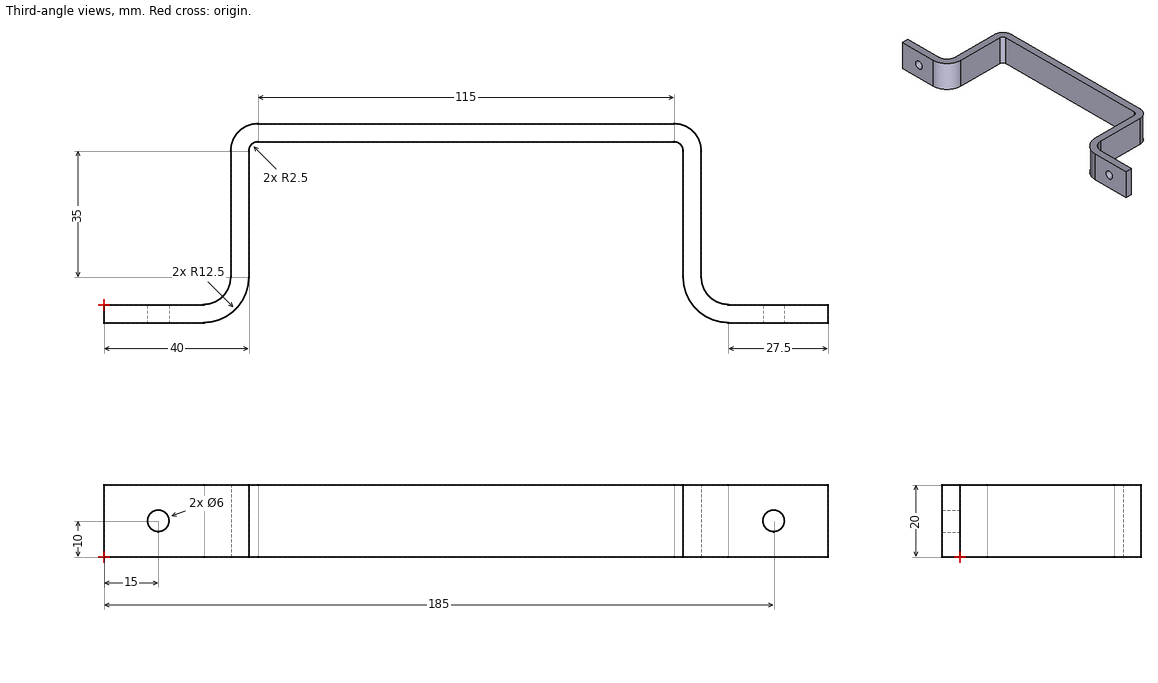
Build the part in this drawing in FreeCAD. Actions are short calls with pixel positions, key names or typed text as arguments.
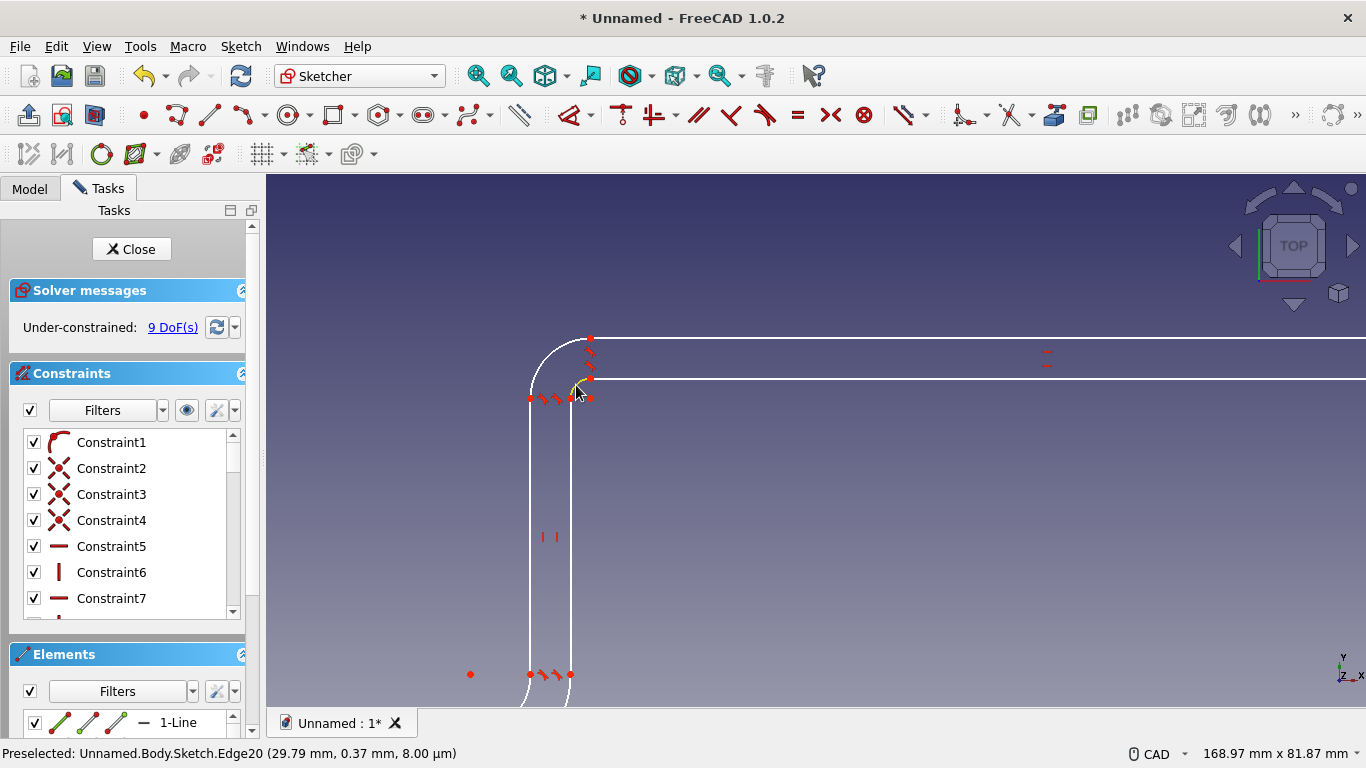
click(576, 384)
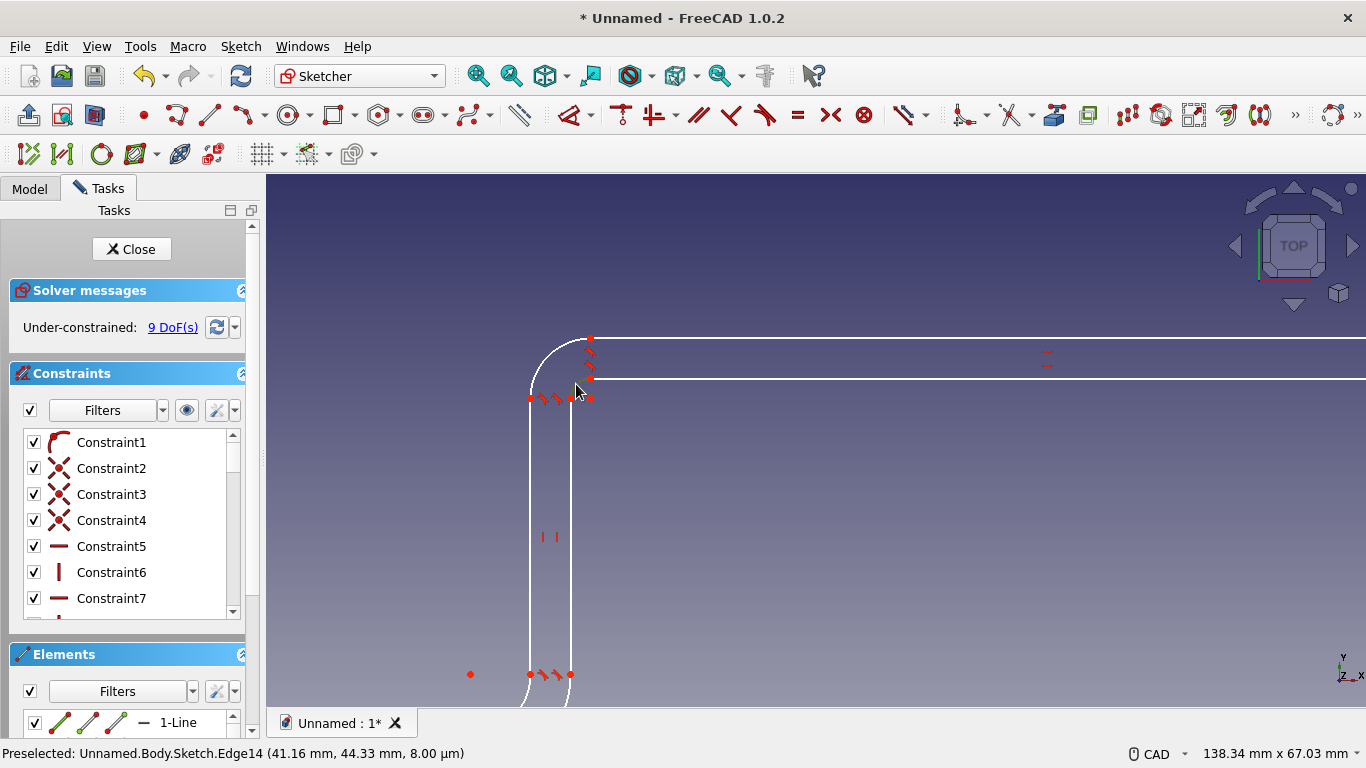
scroll(573, 373, down, 5)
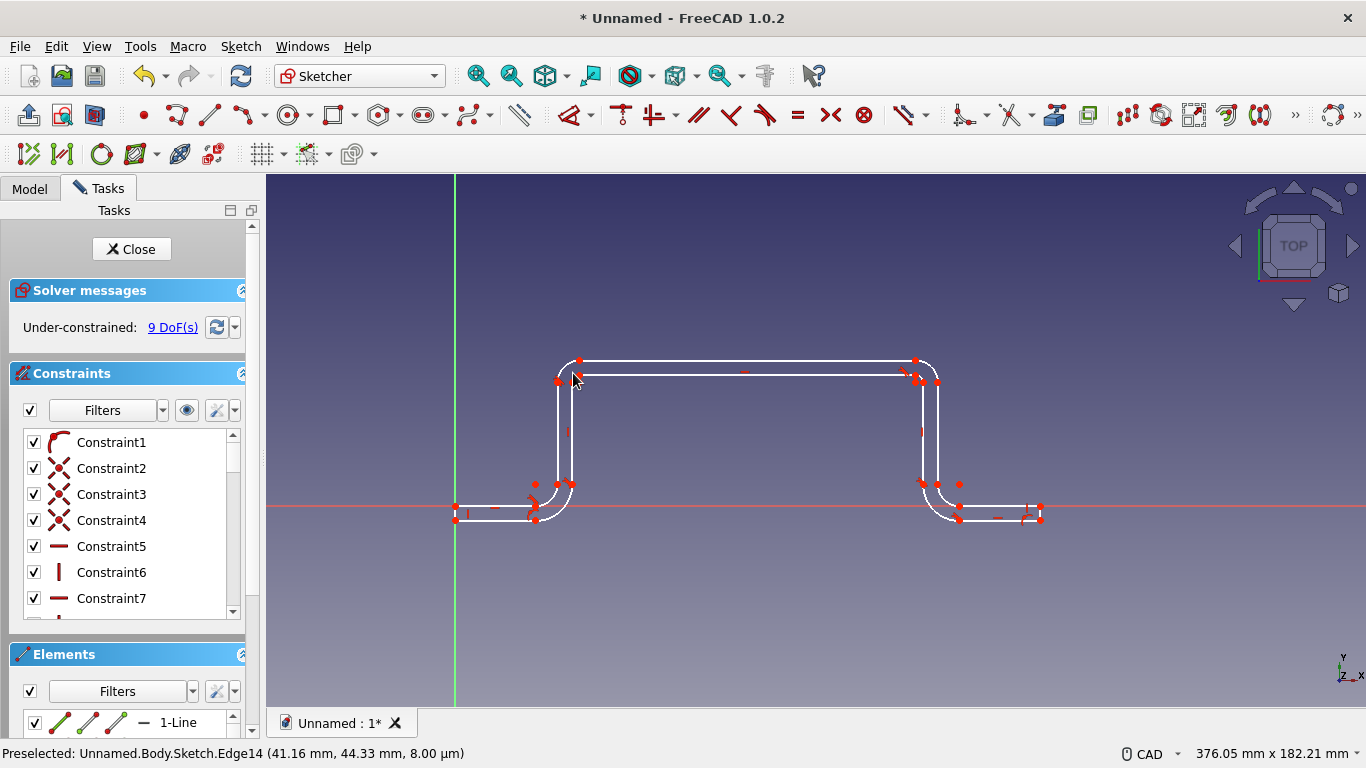
scroll(922, 379, up, 7)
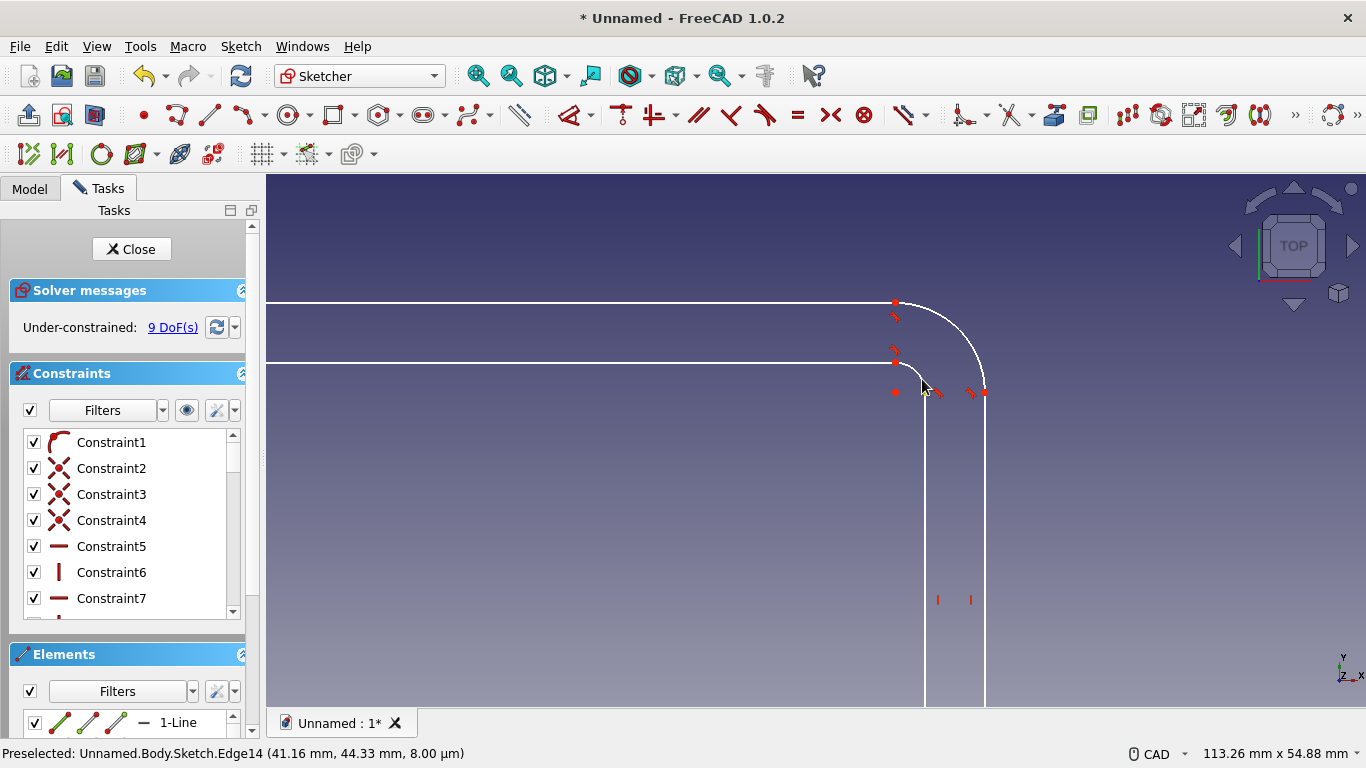
click(922, 379)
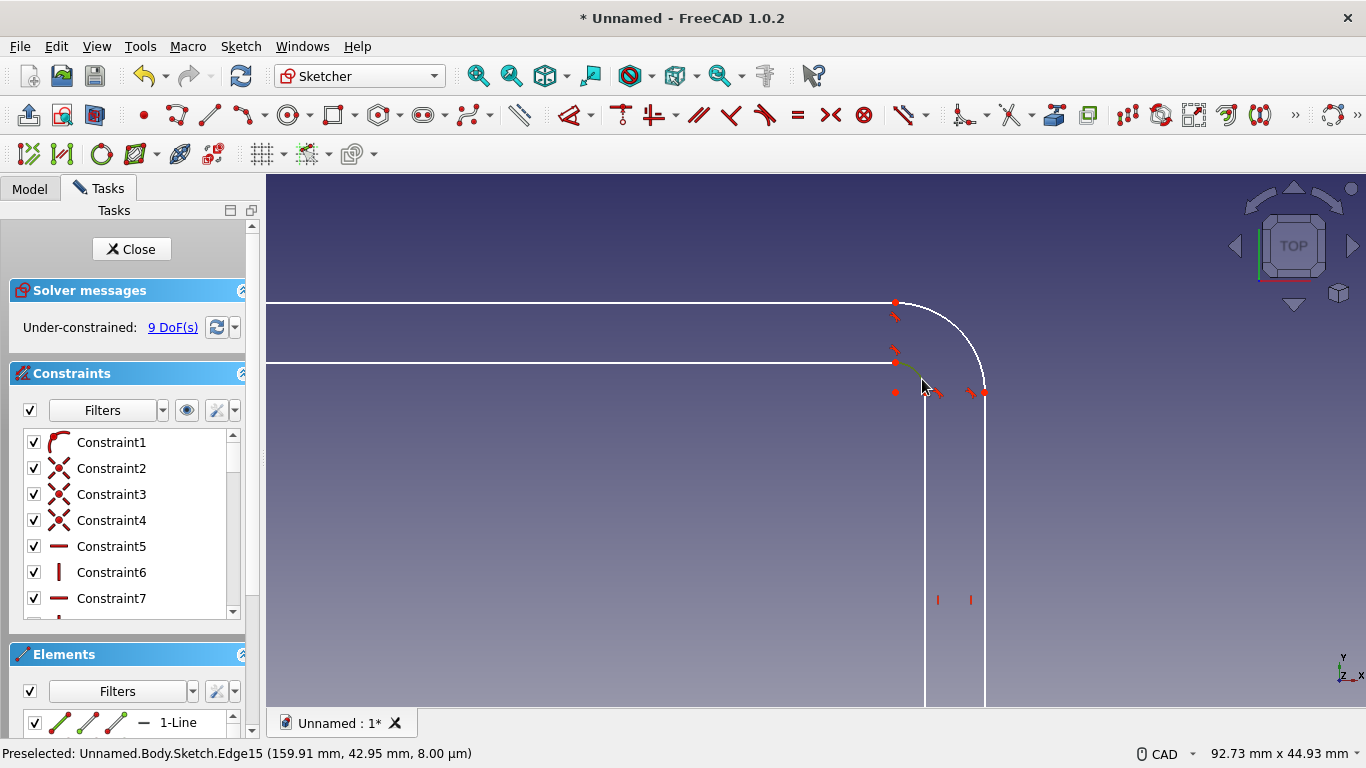
click(798, 116)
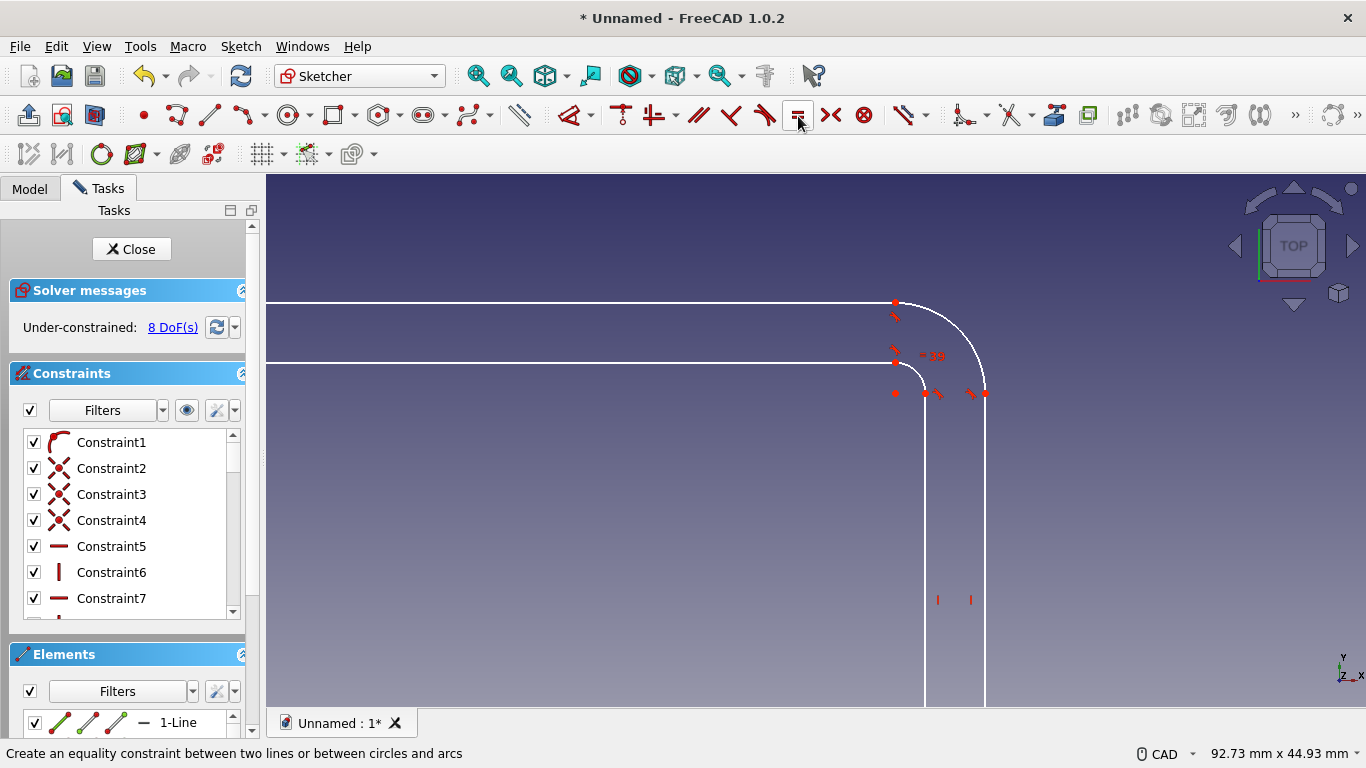
scroll(922, 379, down, 7)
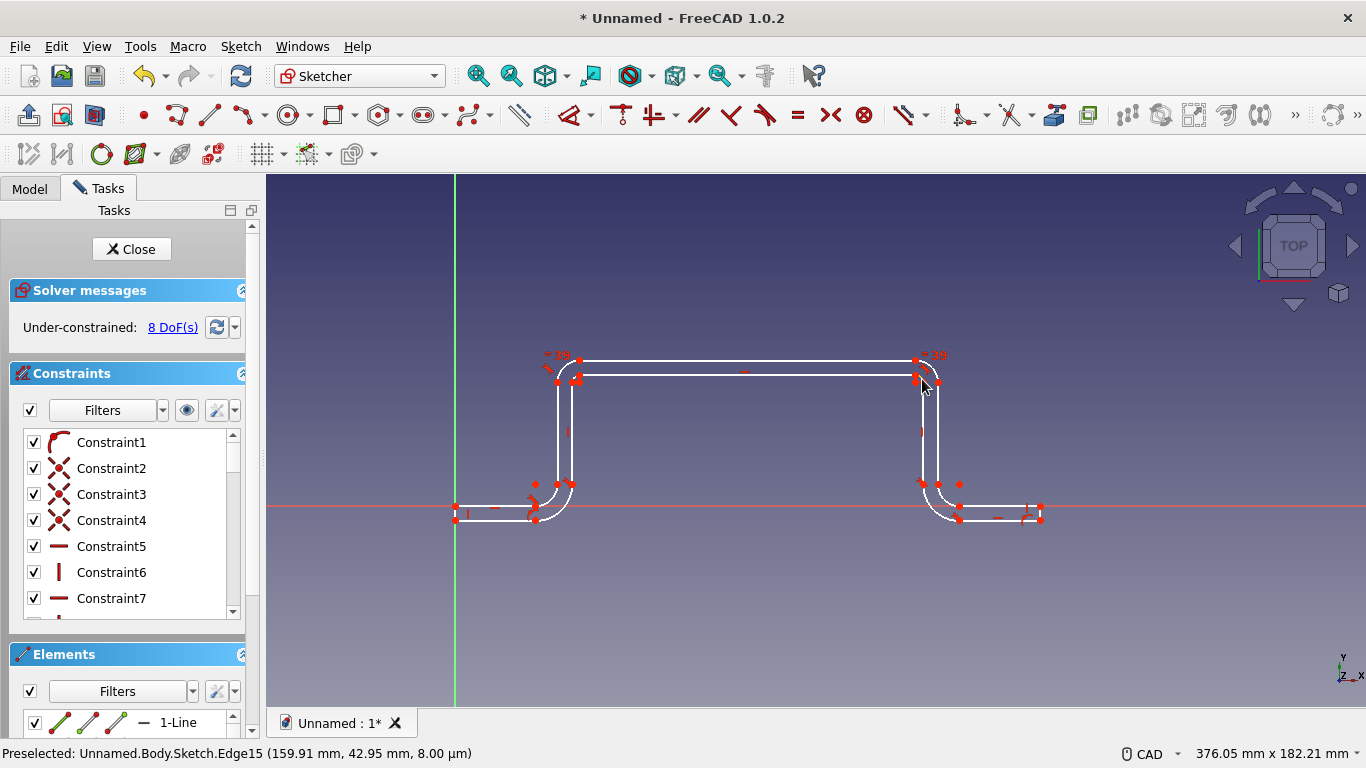
scroll(552, 517, up, 2)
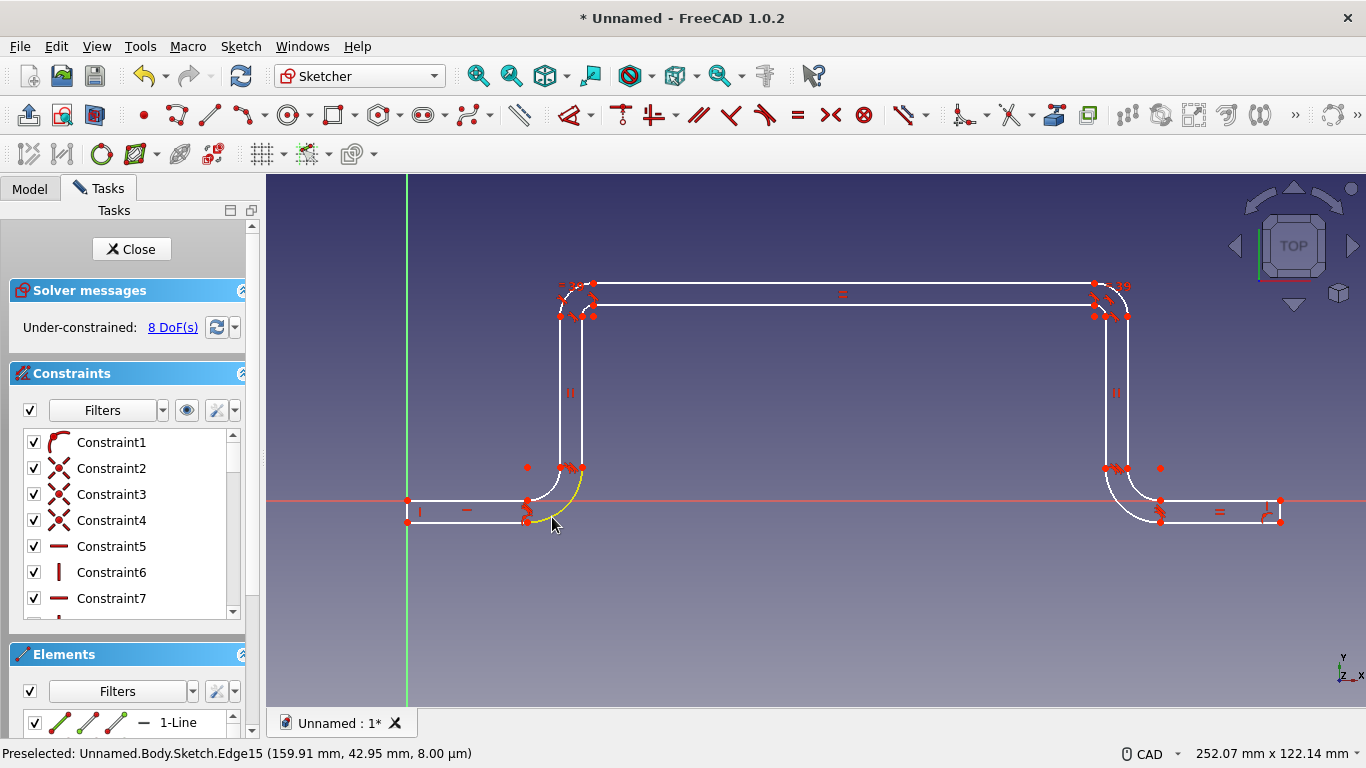
click(552, 517)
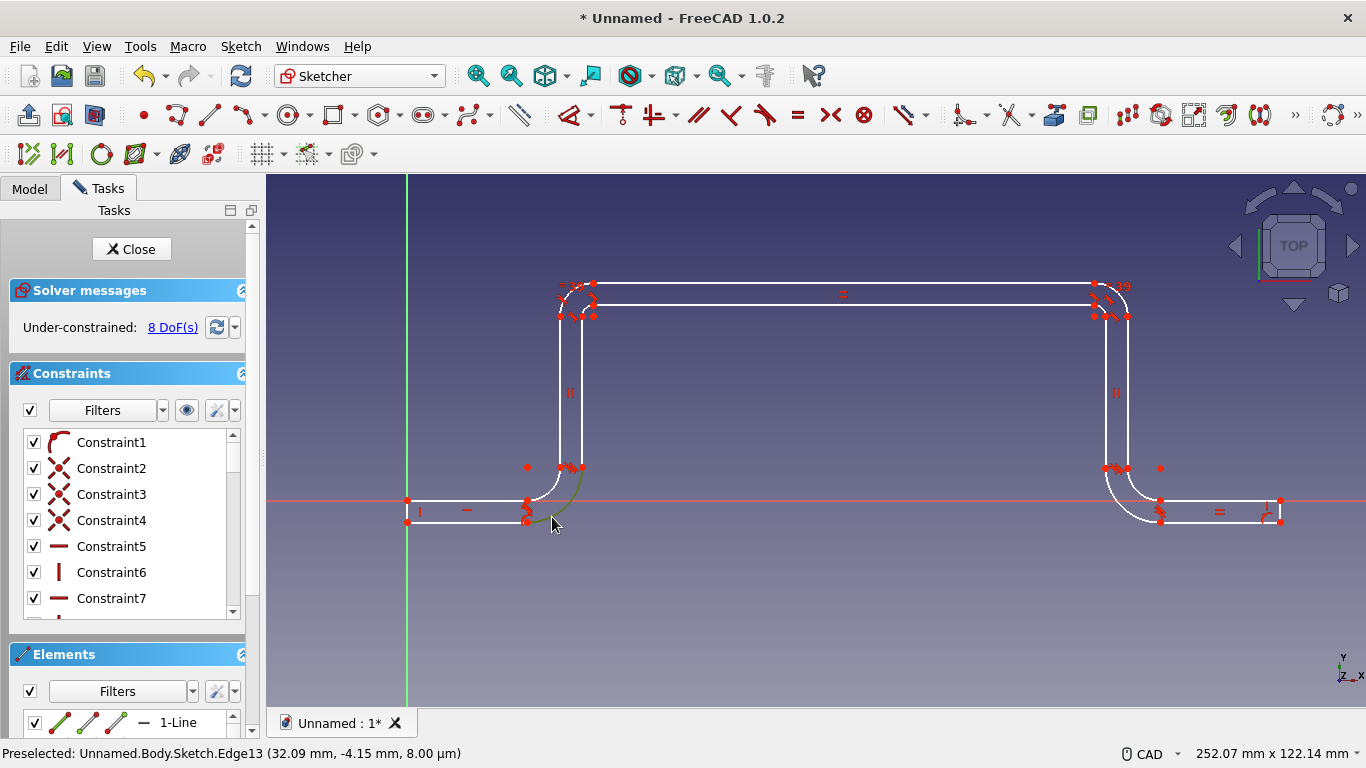
click(1135, 517)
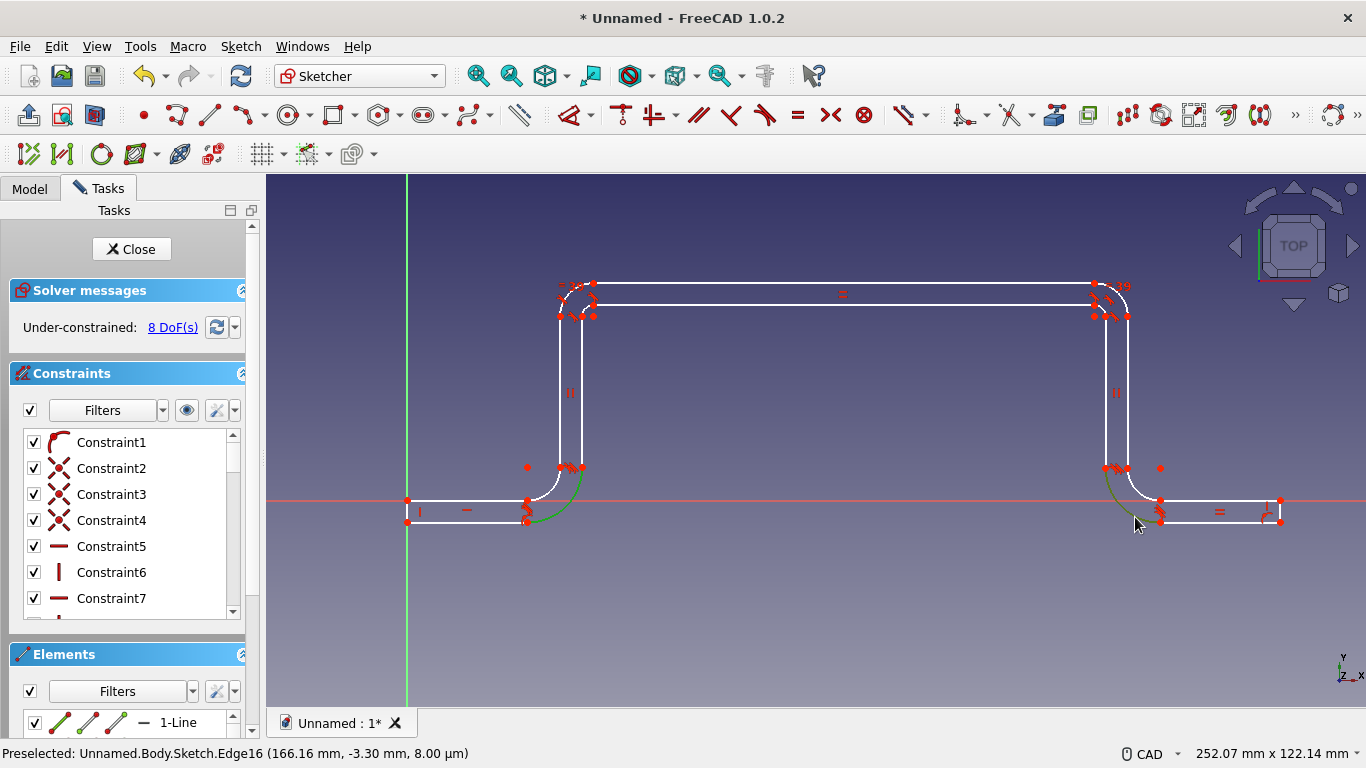
key(e)